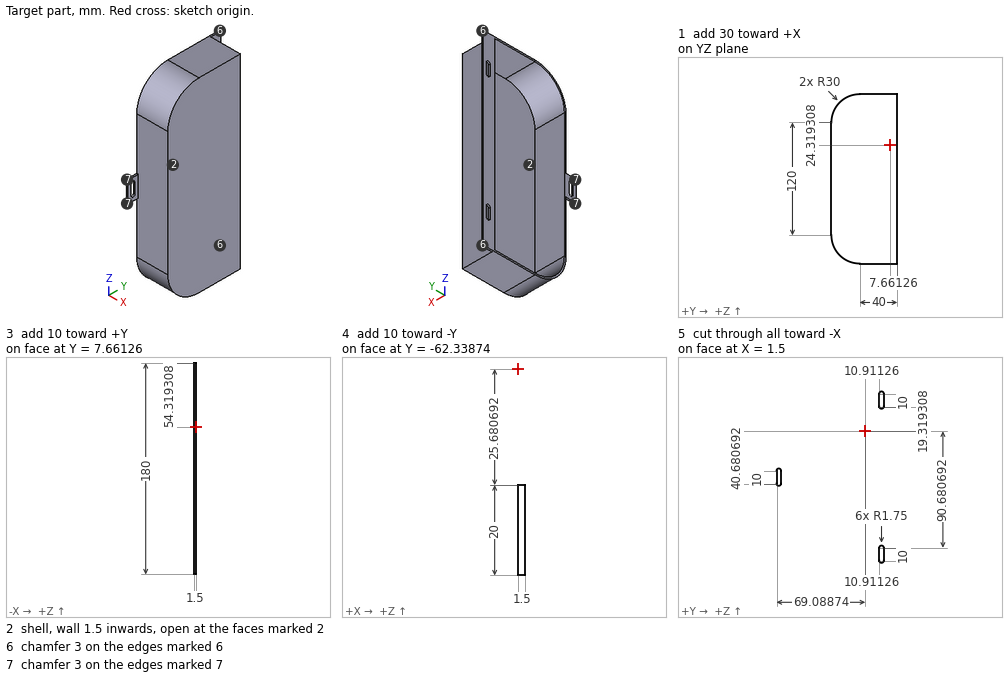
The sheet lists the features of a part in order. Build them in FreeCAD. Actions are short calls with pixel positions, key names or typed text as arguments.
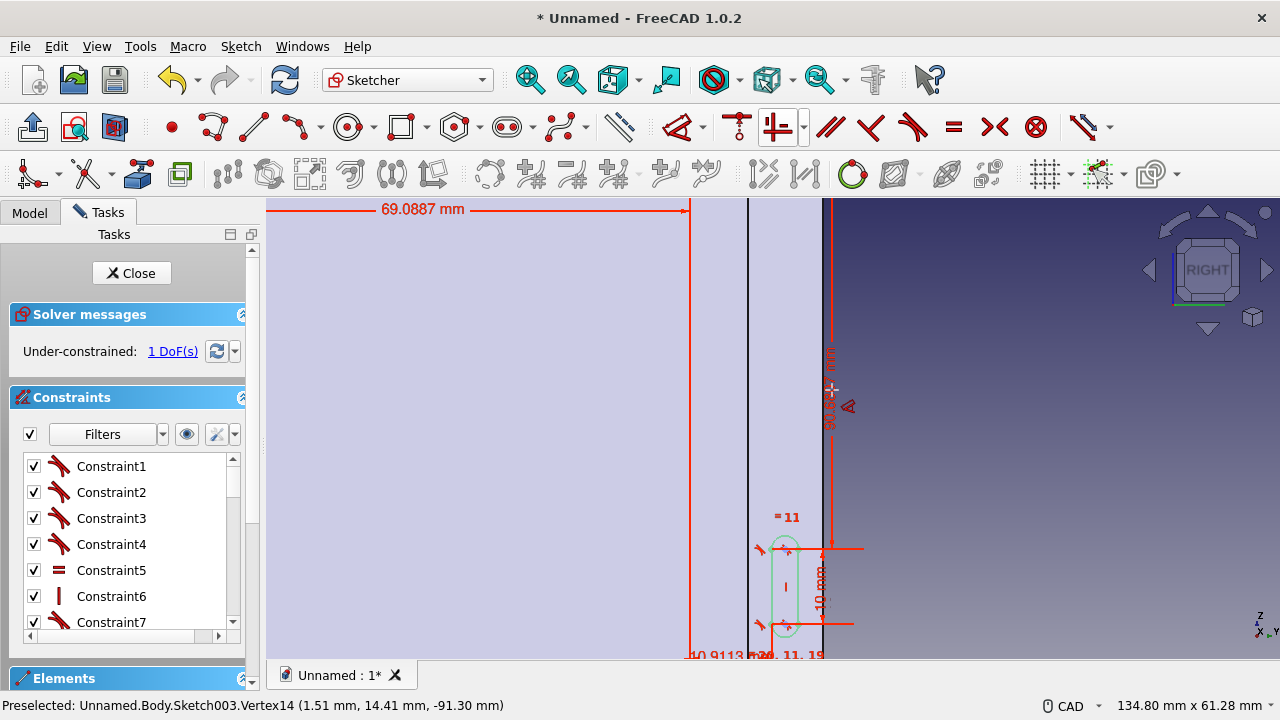
scroll(799, 555, down, 6)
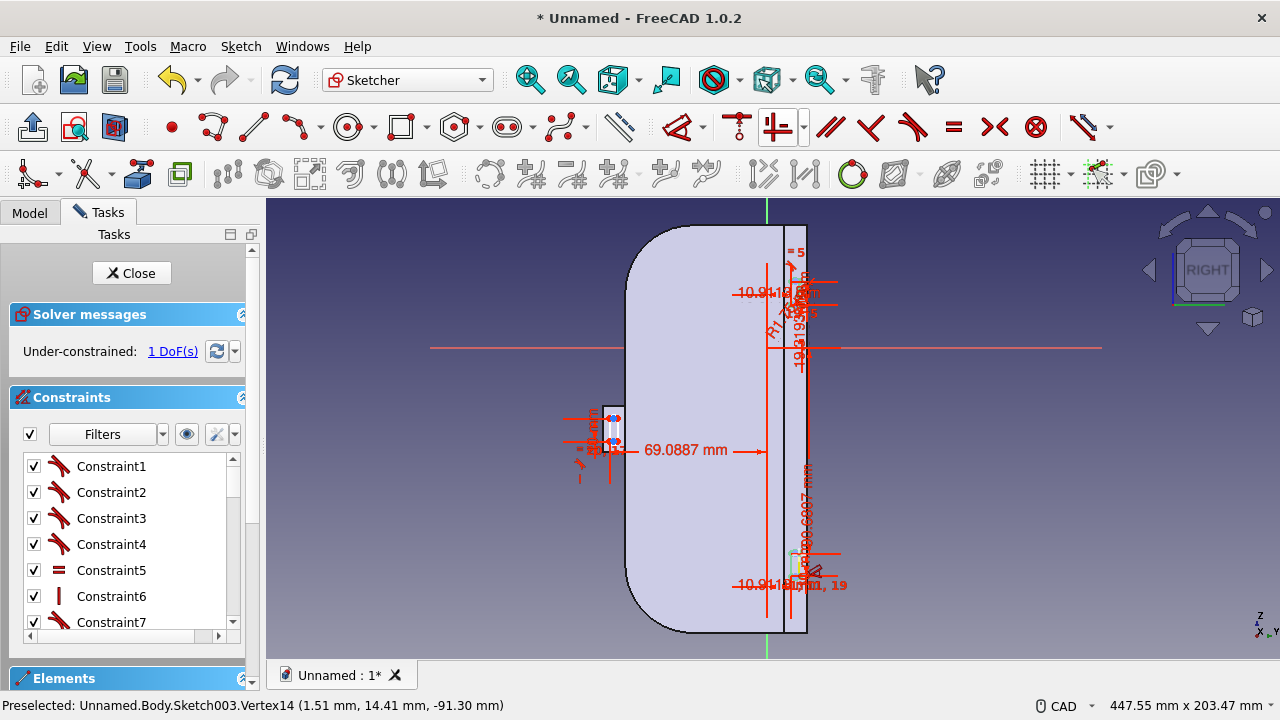
scroll(610, 442, up, 6)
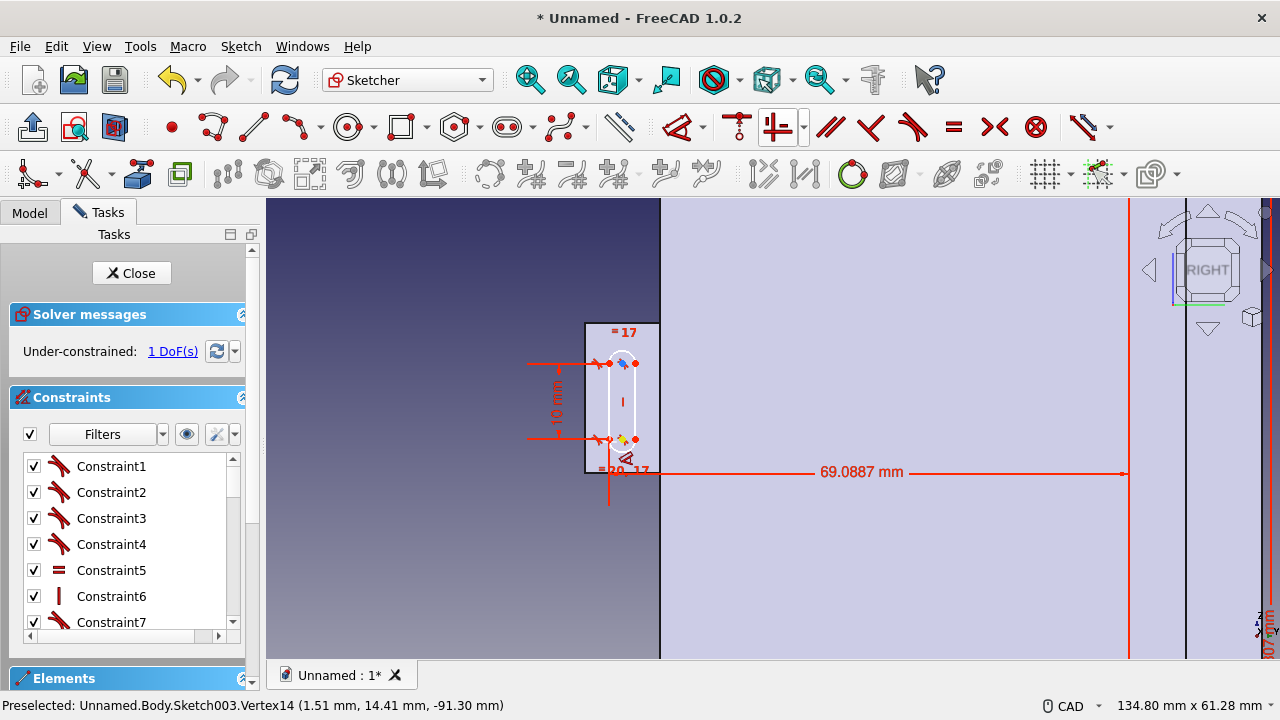
click(609, 439)
click(575, 333)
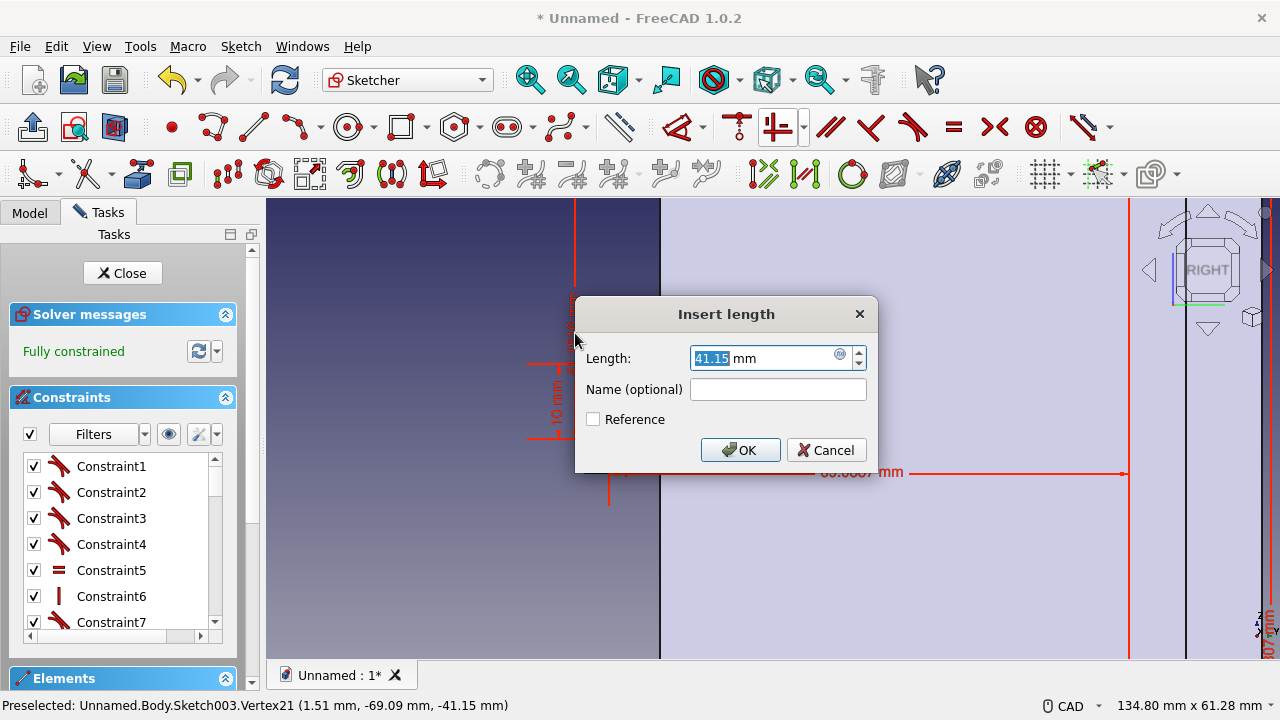
text(40.680692)
key(Return)
key(Escape)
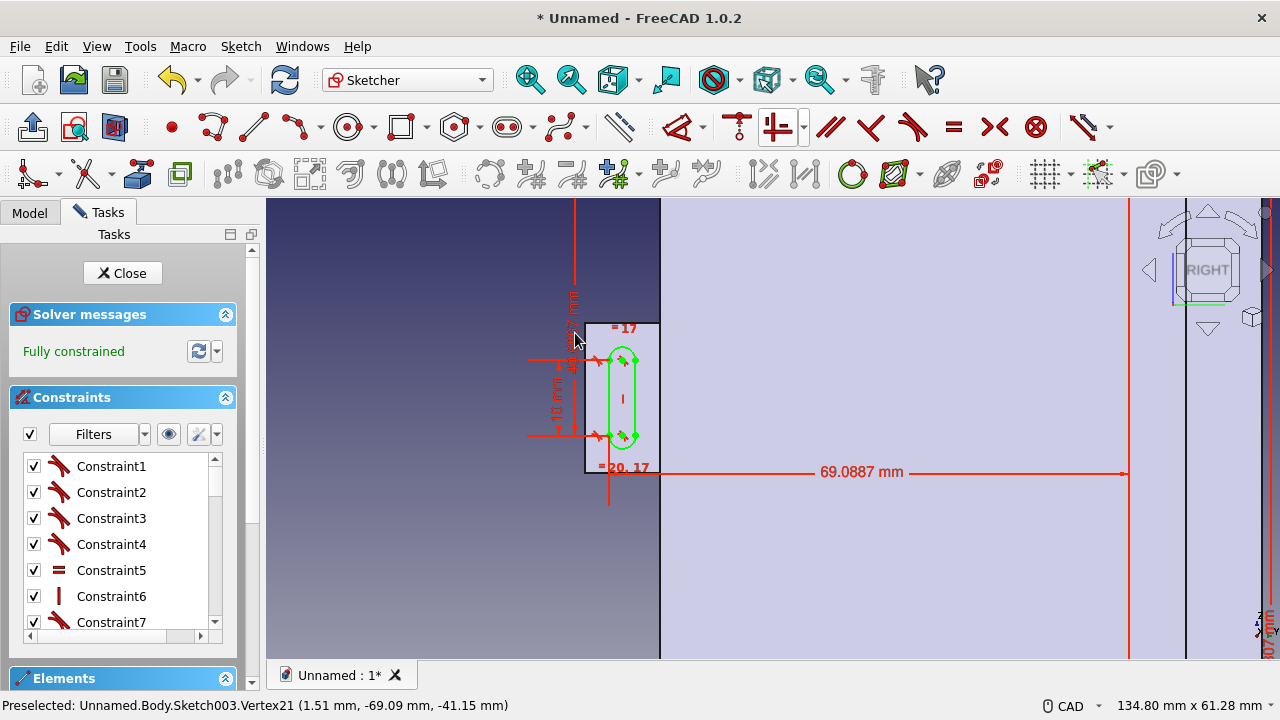
click(123, 273)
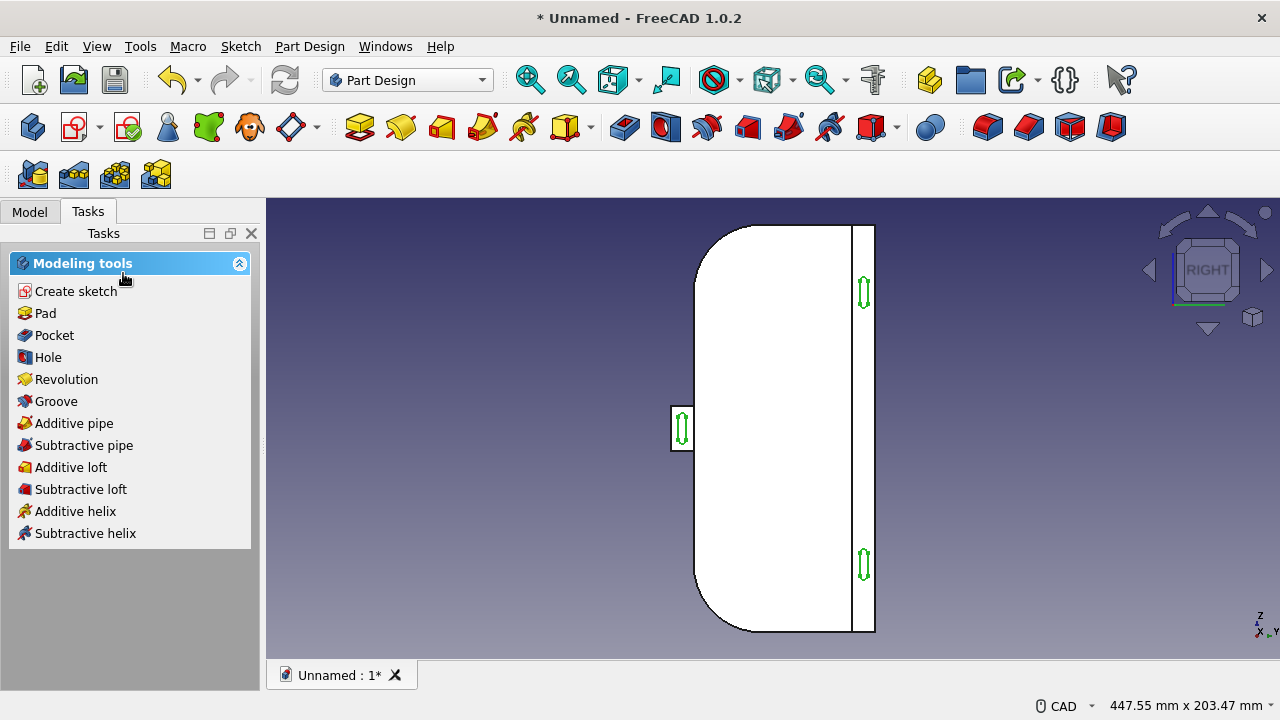
click(625, 128)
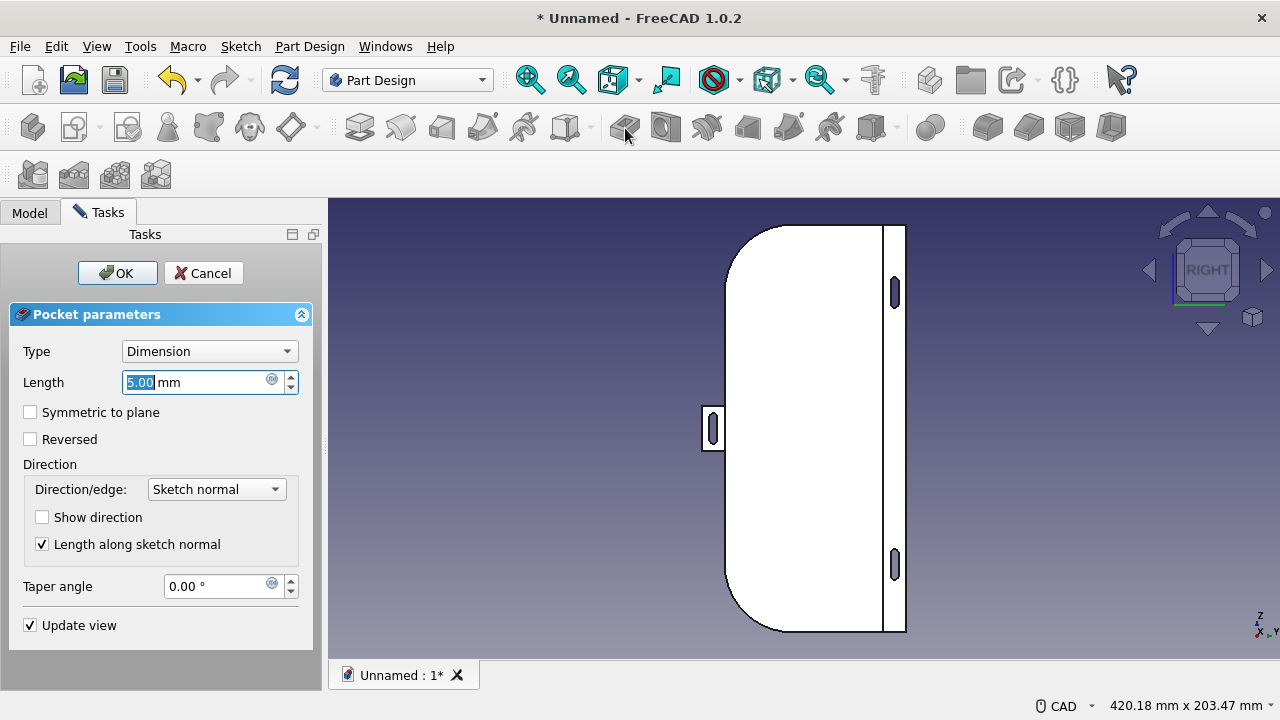
click(210, 352)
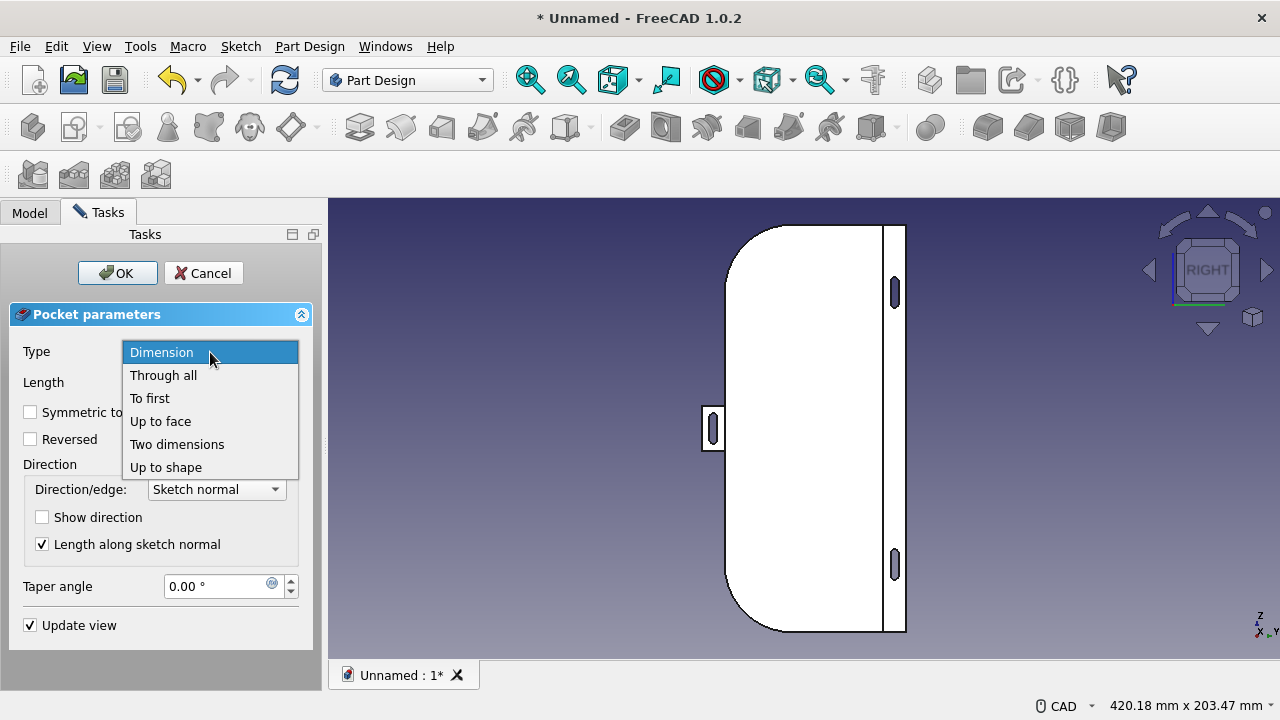
click(208, 376)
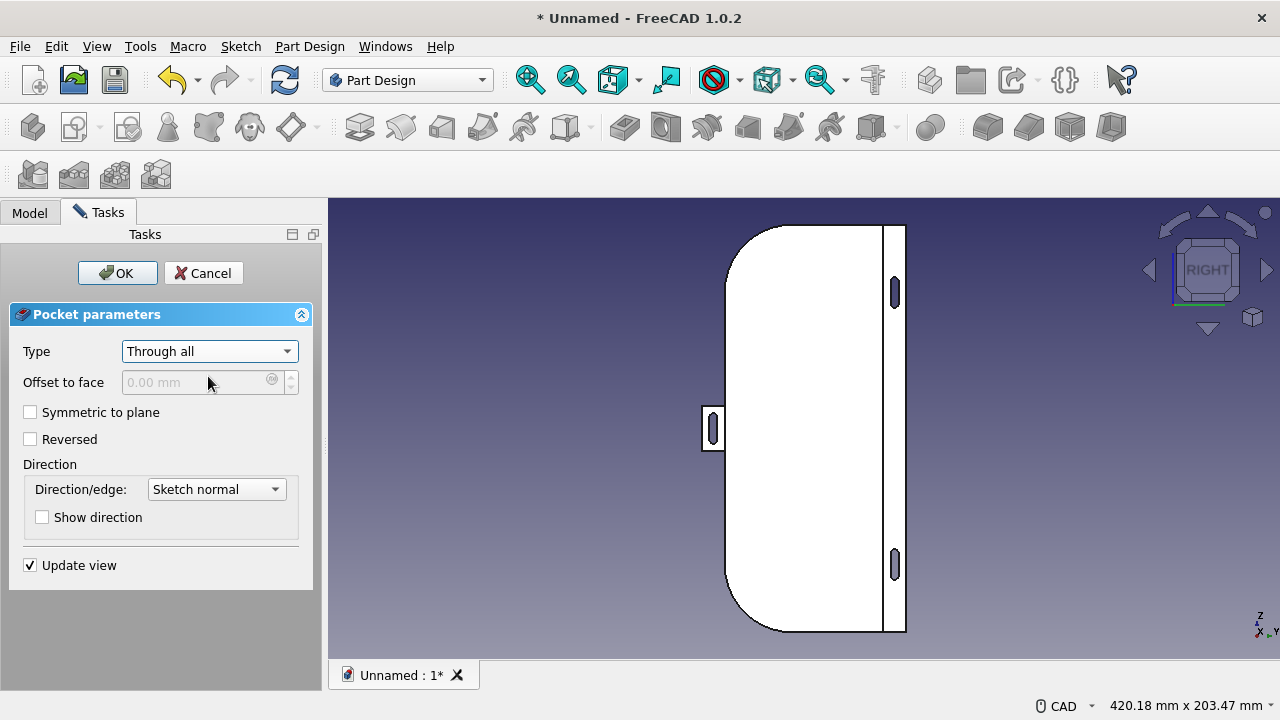
click(118, 273)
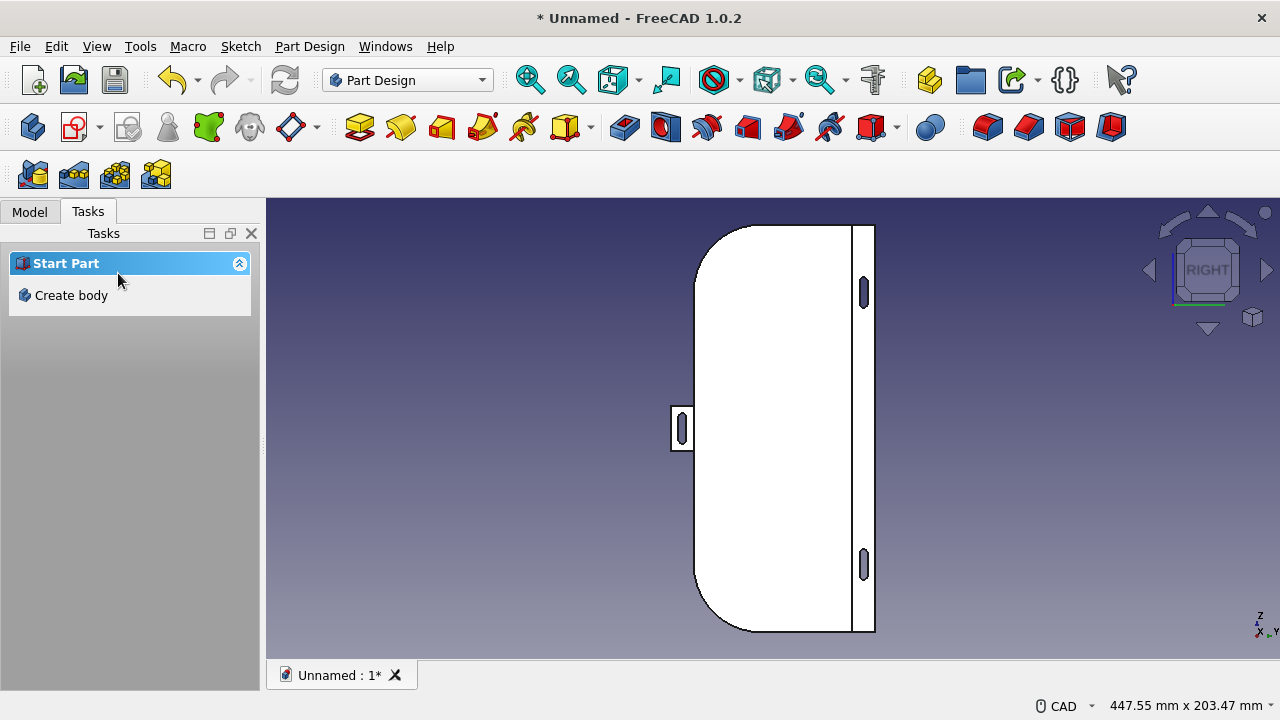
key(0)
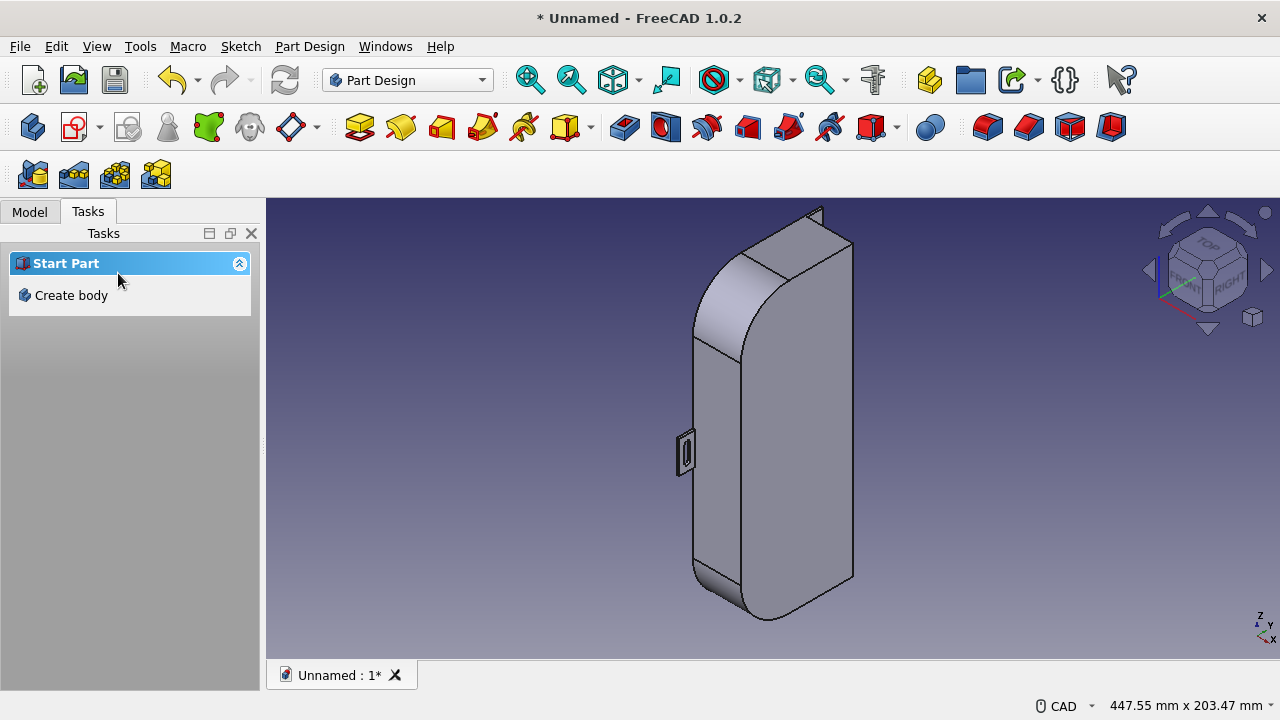
scroll(822, 539, up, 13)